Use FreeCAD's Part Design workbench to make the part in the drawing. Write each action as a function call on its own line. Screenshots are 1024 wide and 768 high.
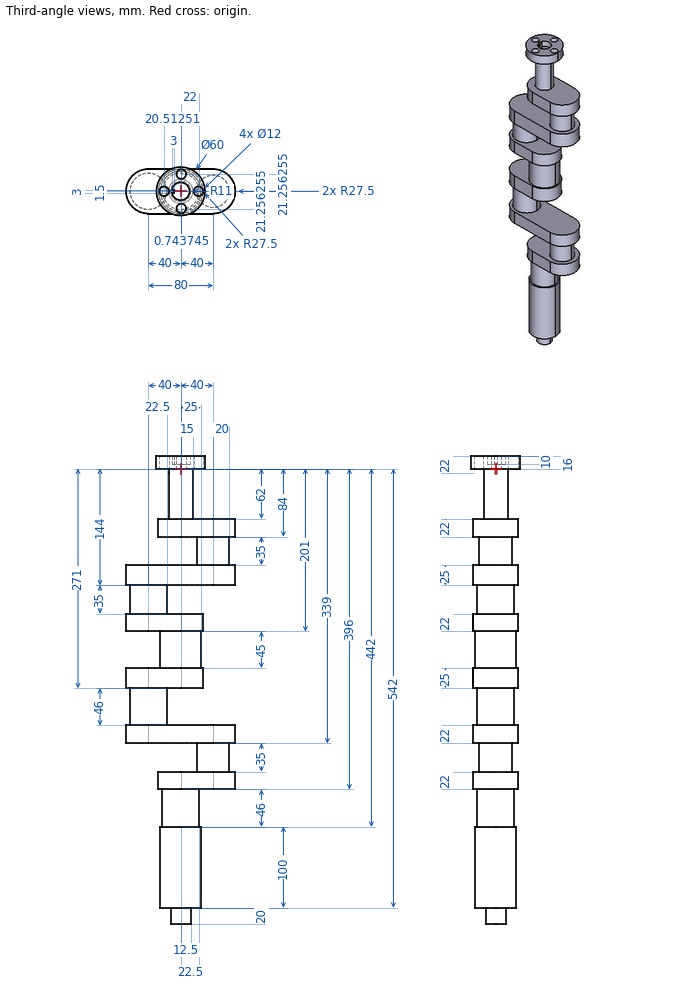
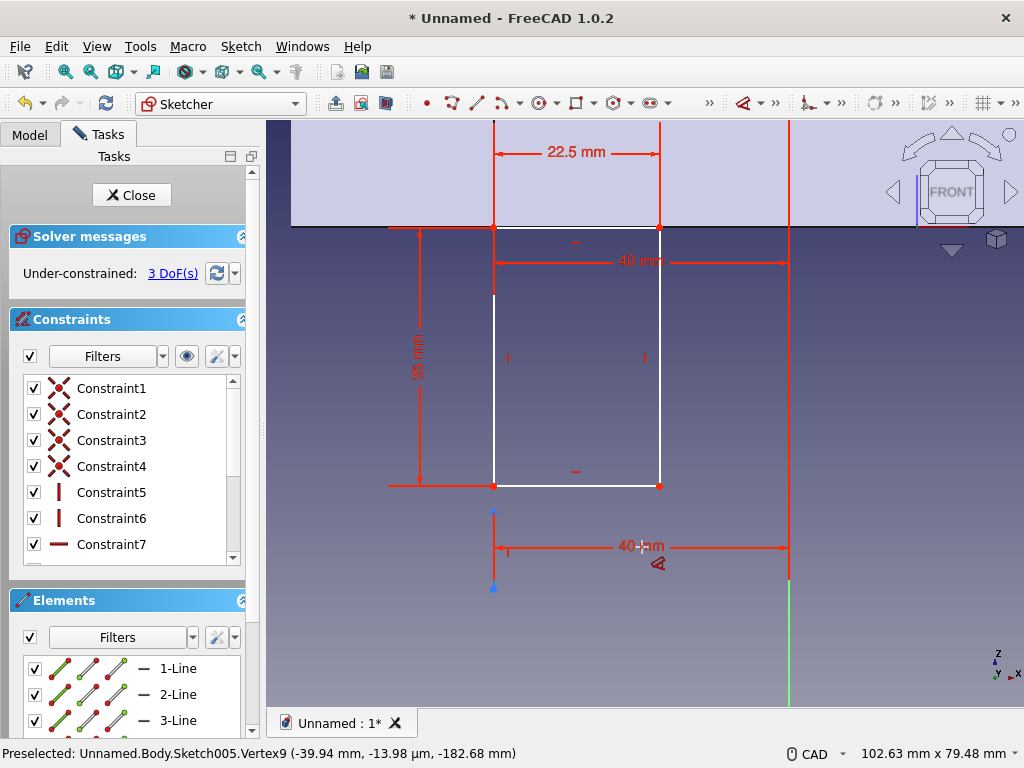
click(494, 228)
click(823, 188)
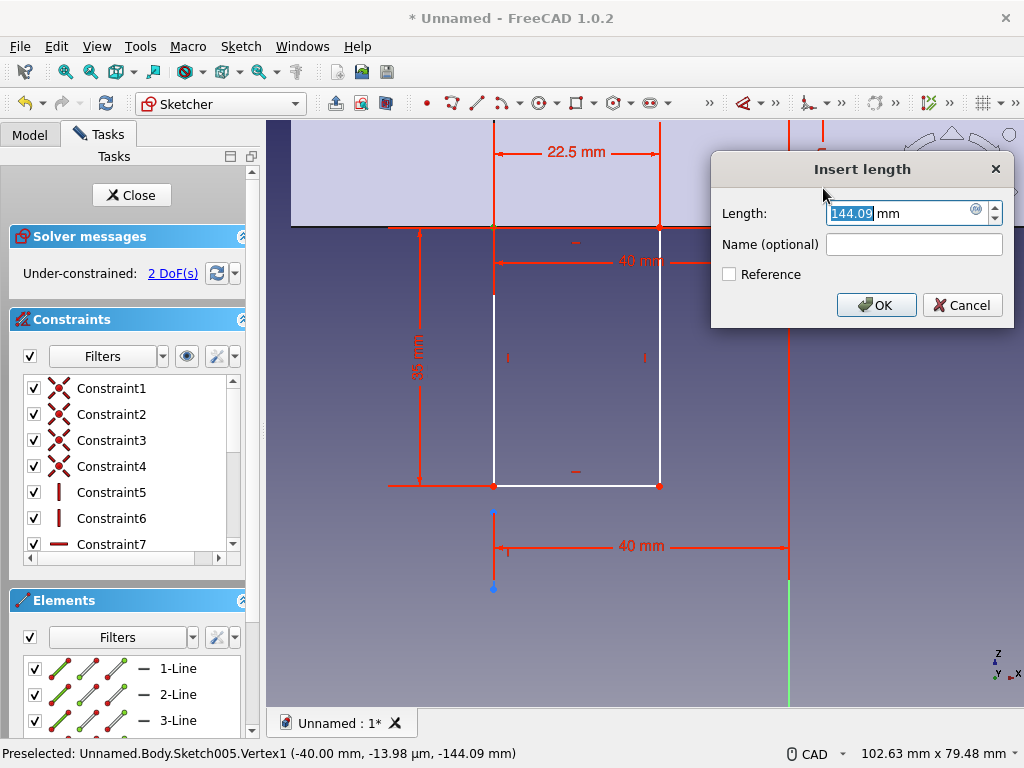
text(144)
key(Return)
key(Escape)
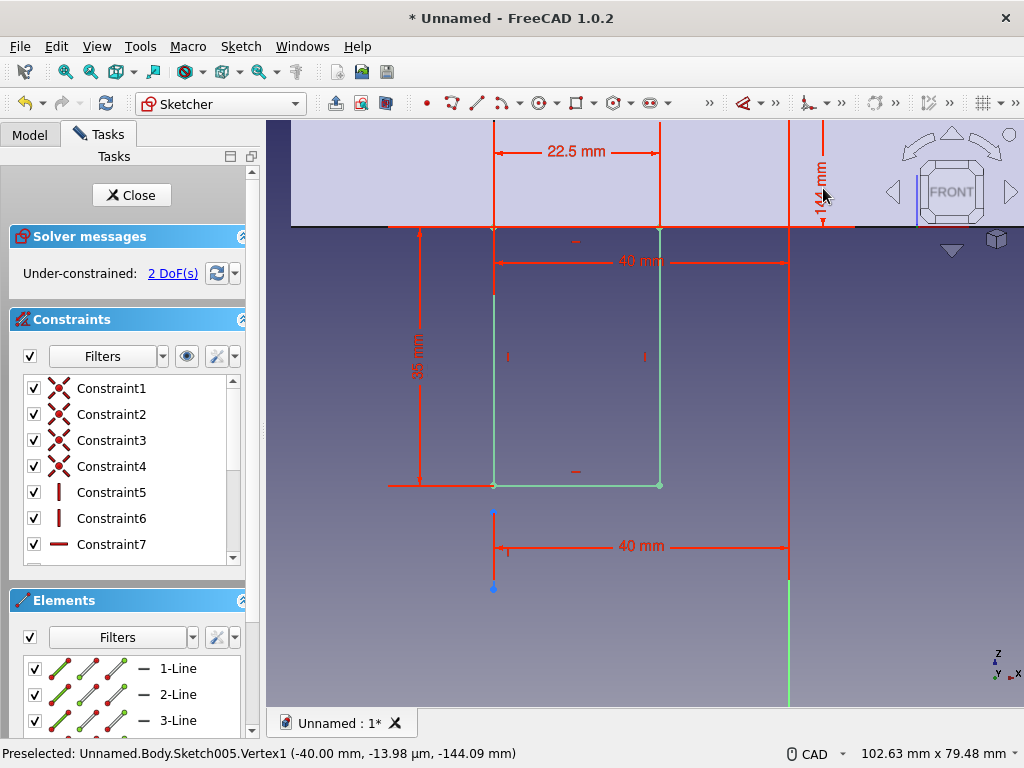
click(132, 195)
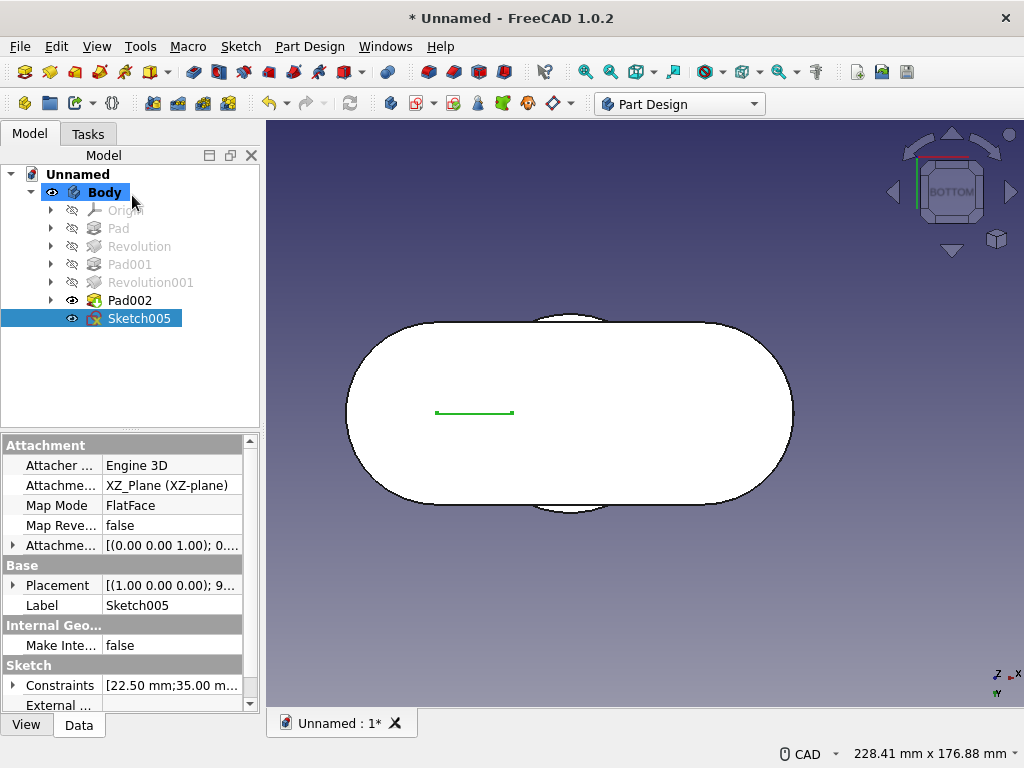
click(50, 72)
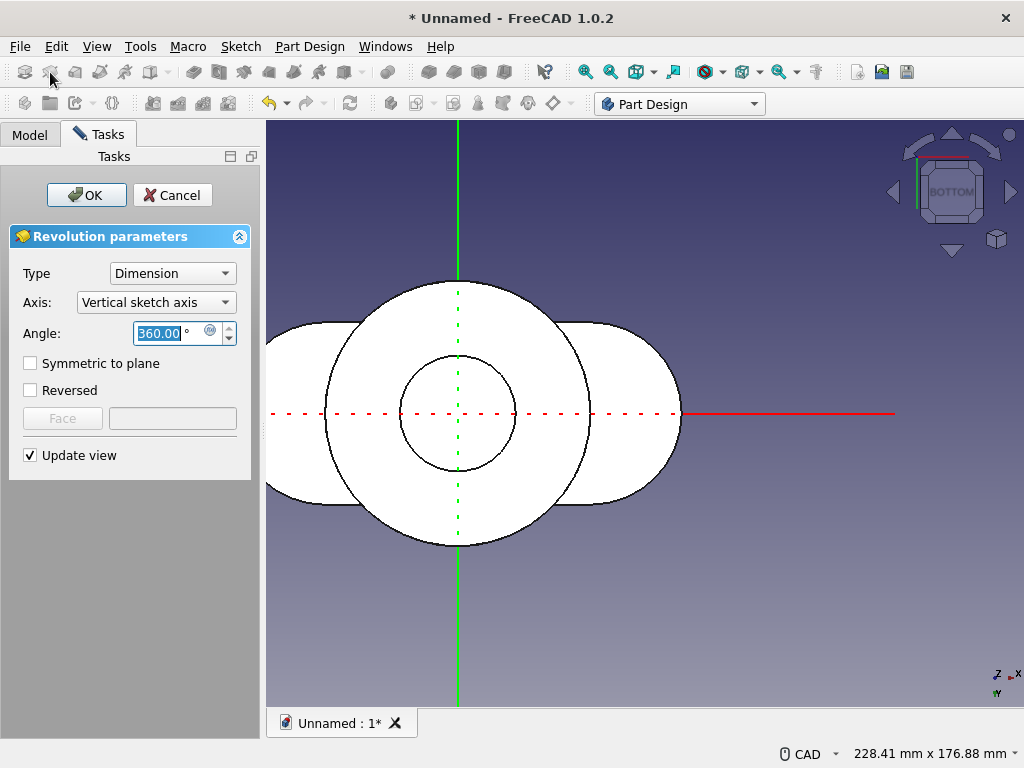
click(157, 302)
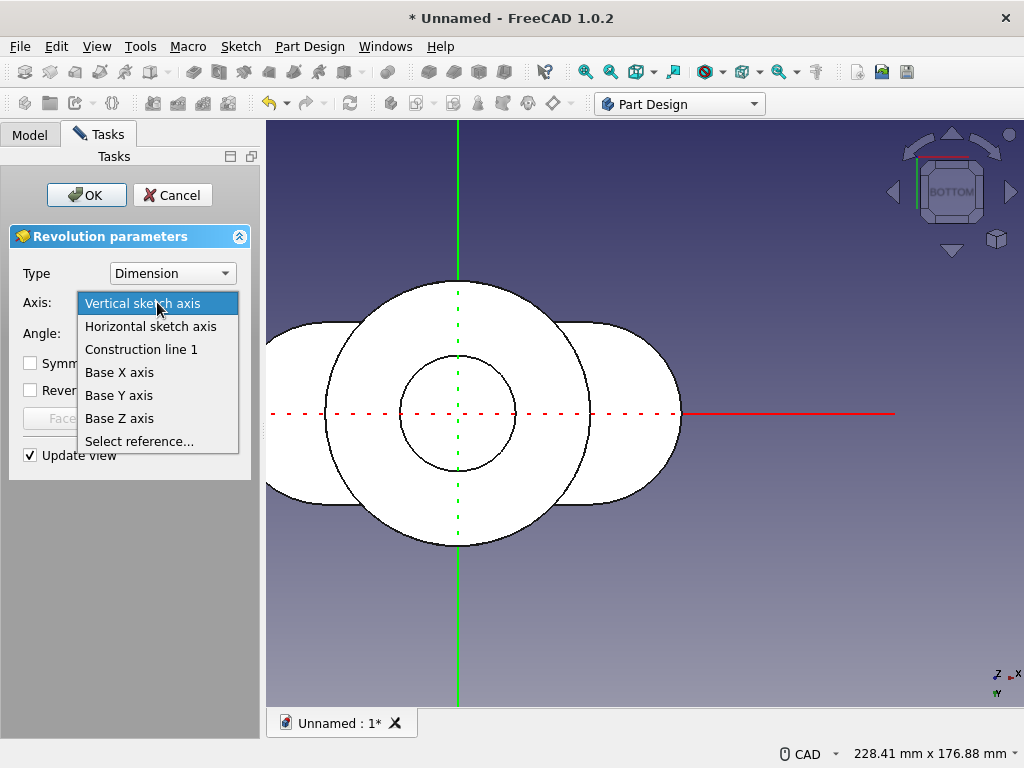
click(156, 350)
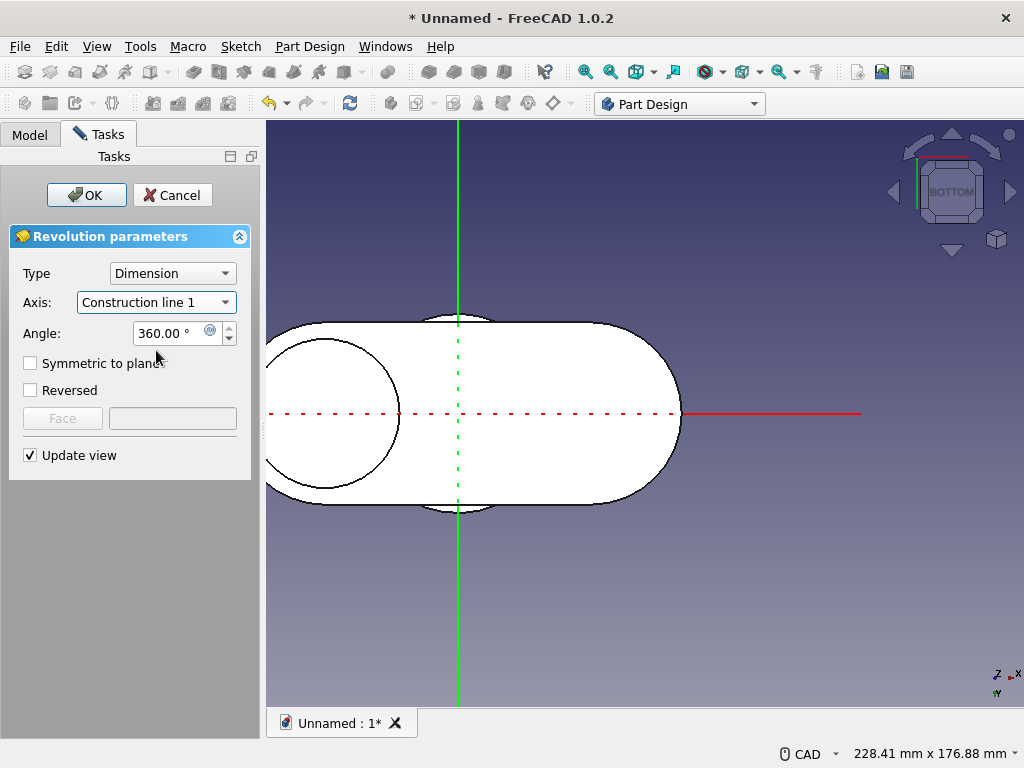
click(87, 195)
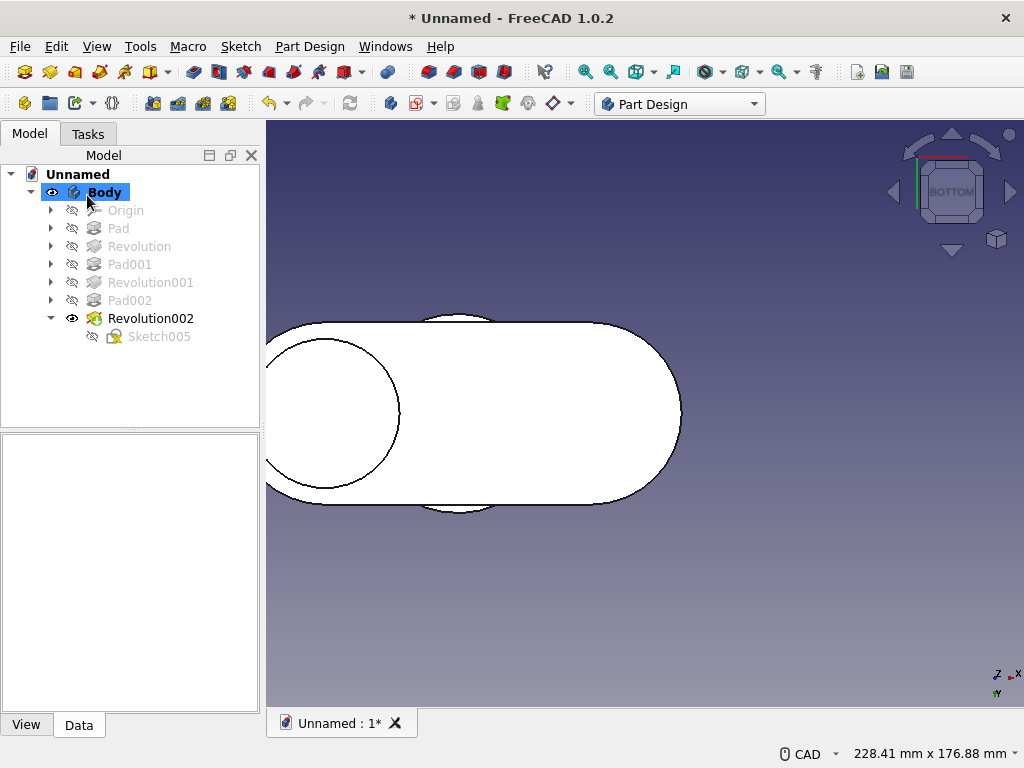
key(v)
key(f)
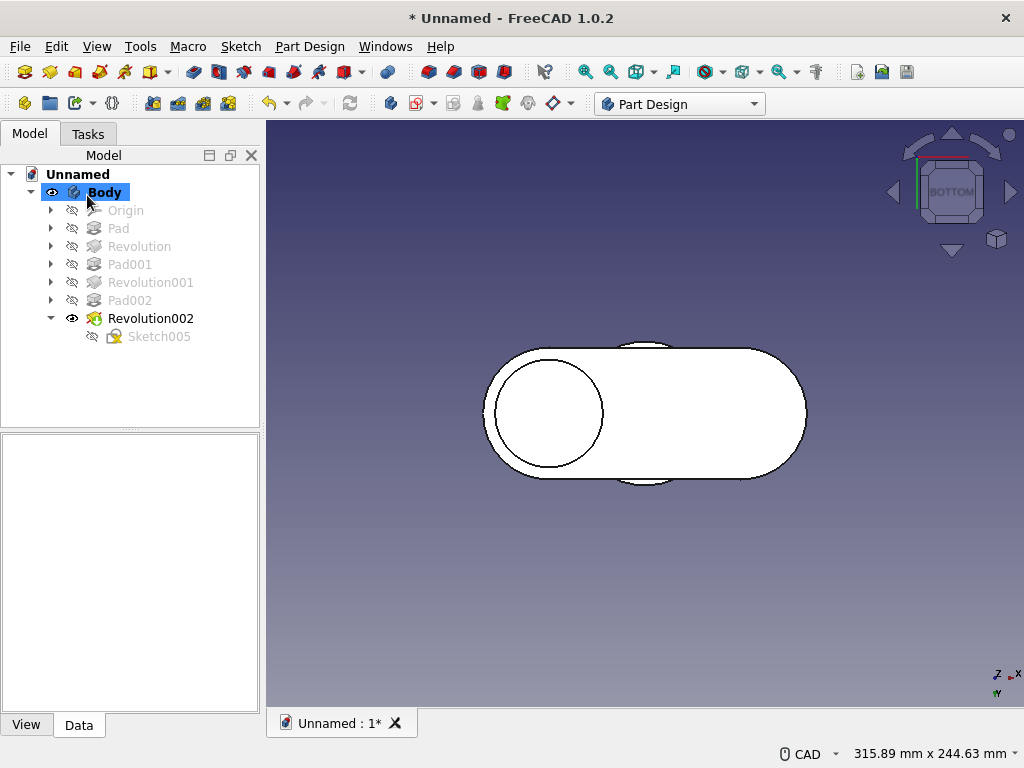
click(549, 412)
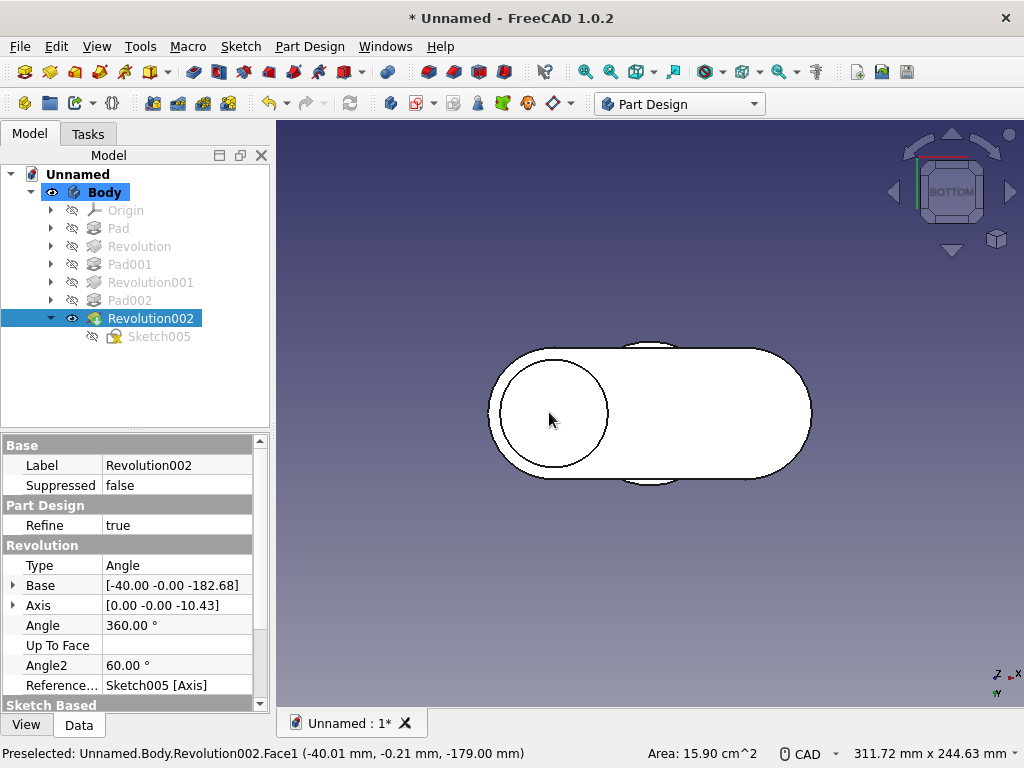
click(416, 104)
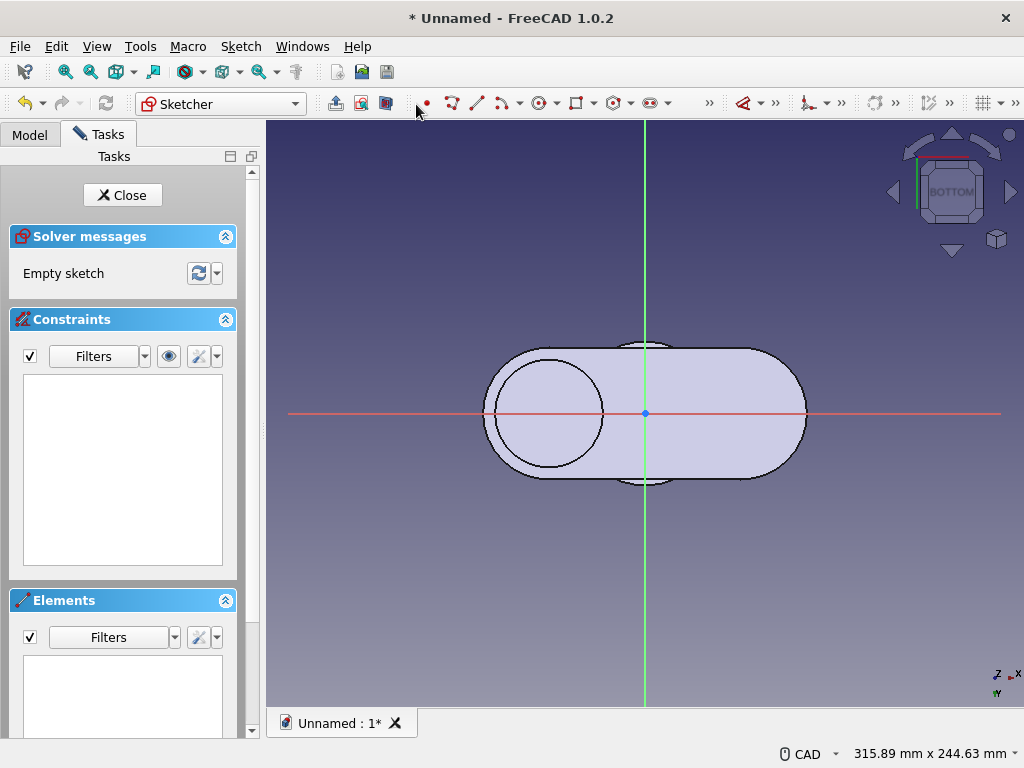
scroll(622, 413, up, 3)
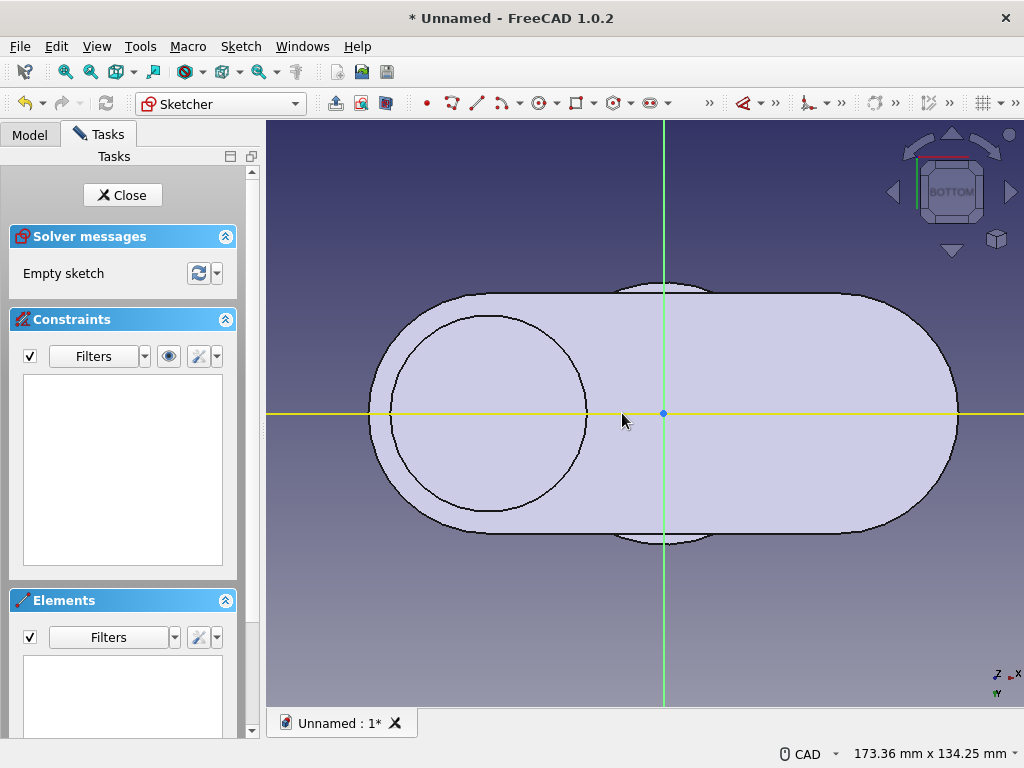
key(g)
key(s)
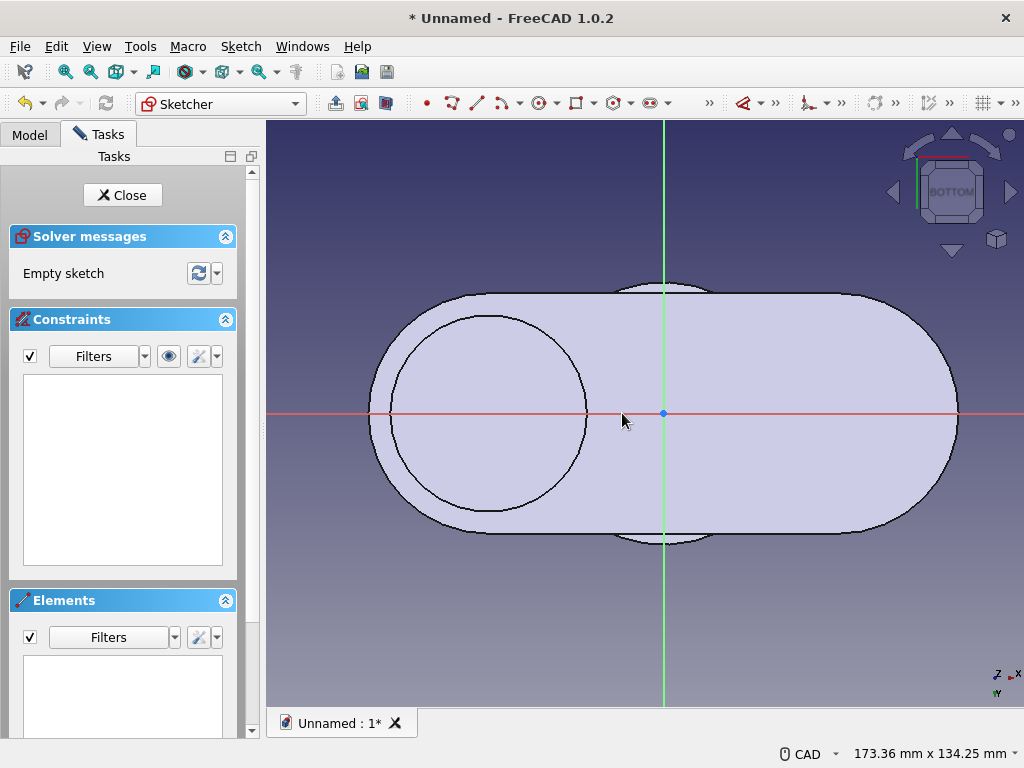
click(664, 413)